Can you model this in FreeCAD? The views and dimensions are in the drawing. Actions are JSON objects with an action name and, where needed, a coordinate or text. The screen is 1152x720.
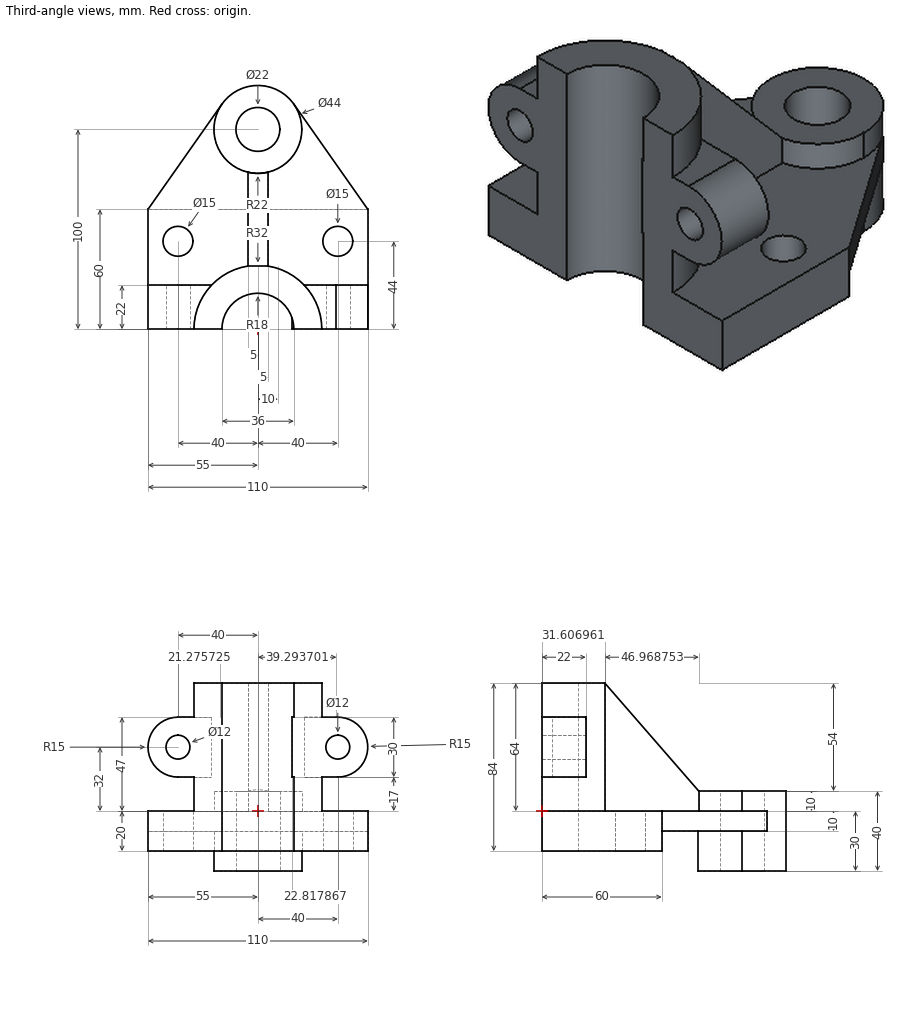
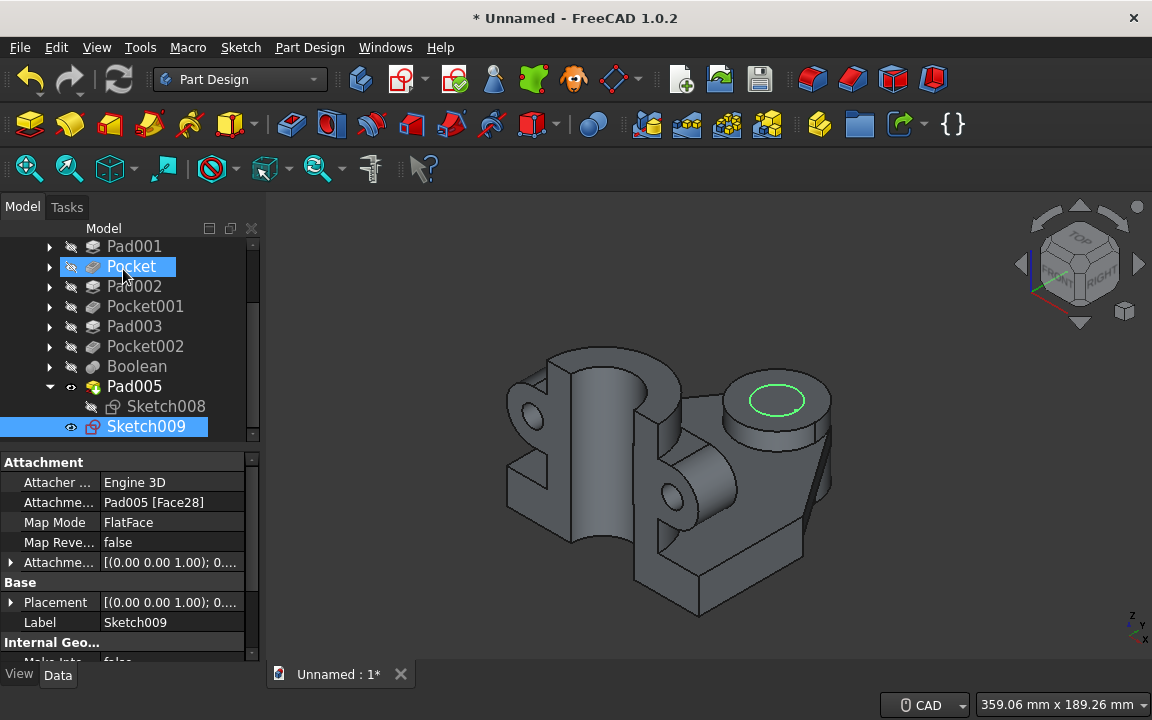
{"action": "left_click", "coordinate": [292, 124]}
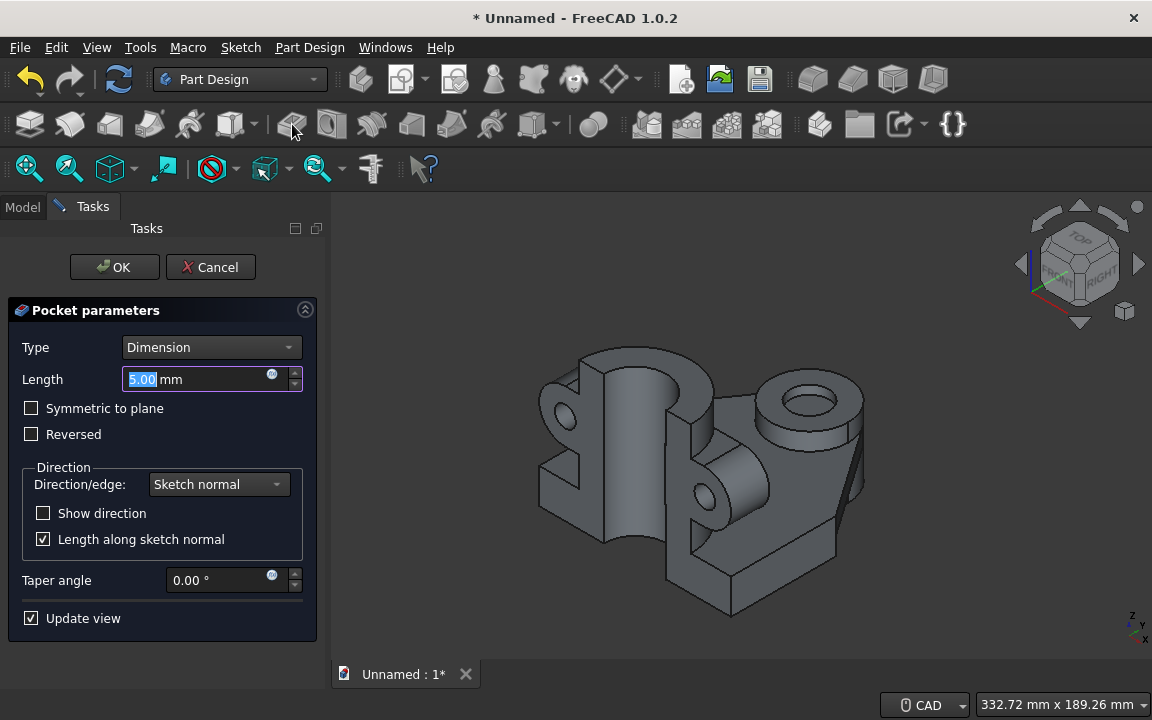
{"action": "type", "text": "40"}
{"action": "key", "text": "Tab"}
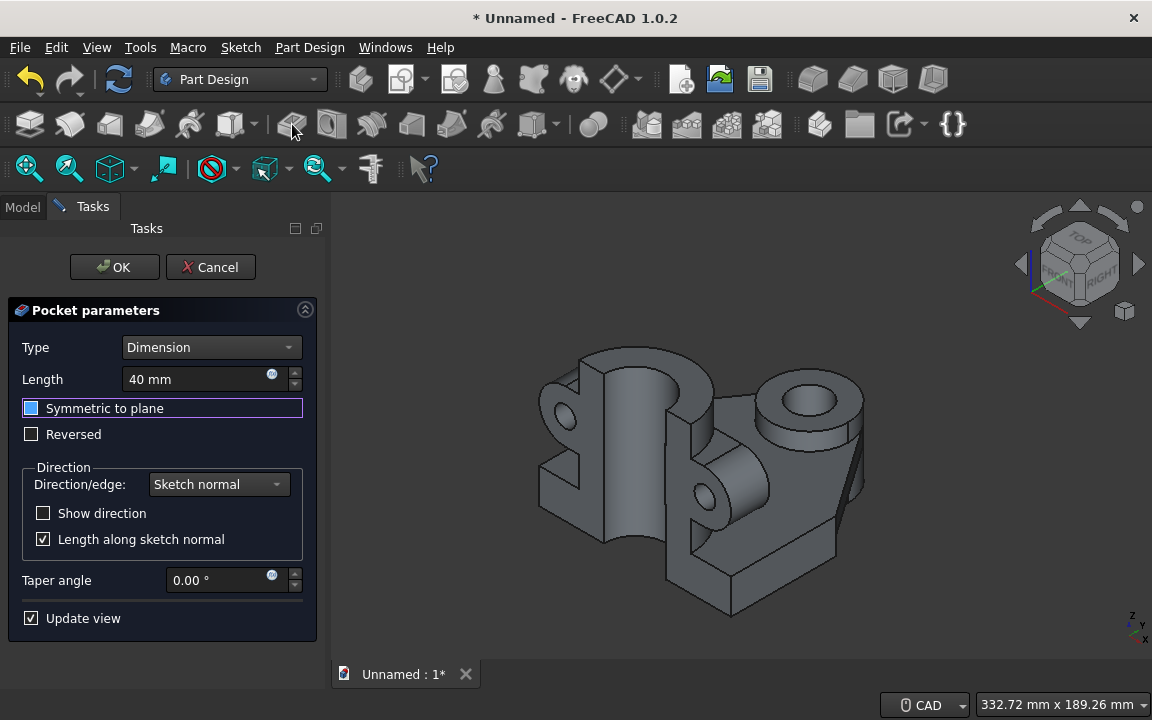
{"action": "left_click", "coordinate": [115, 267]}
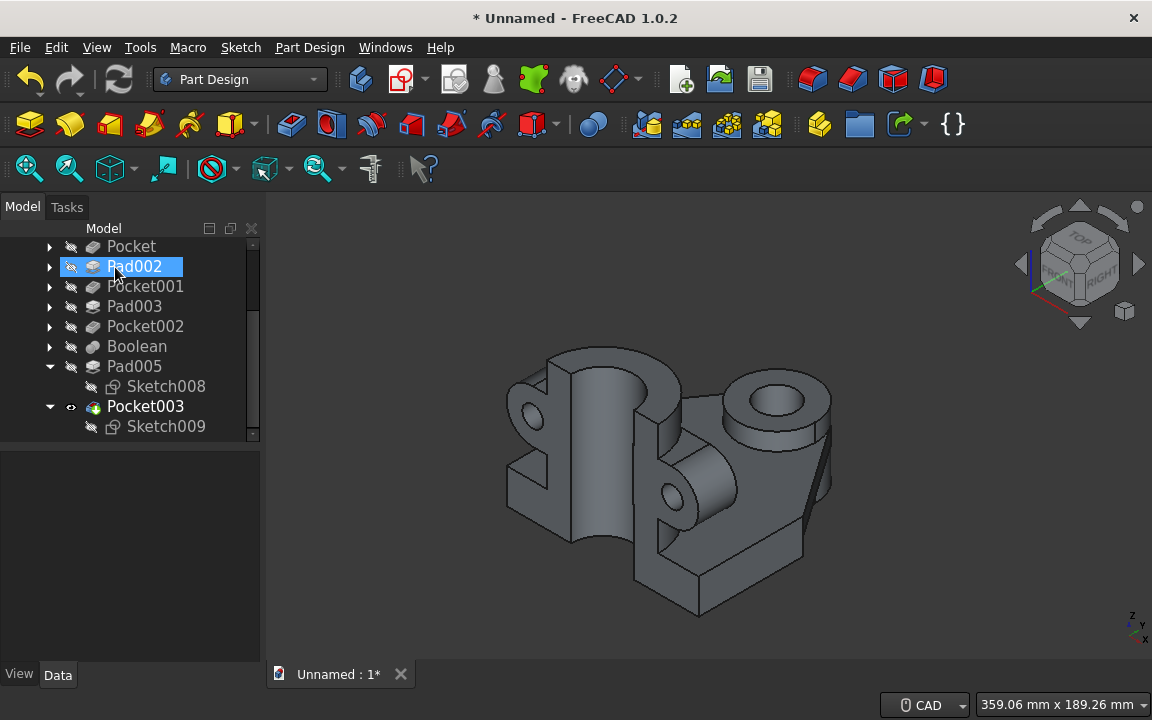
{"action": "left_click", "coordinate": [756, 495]}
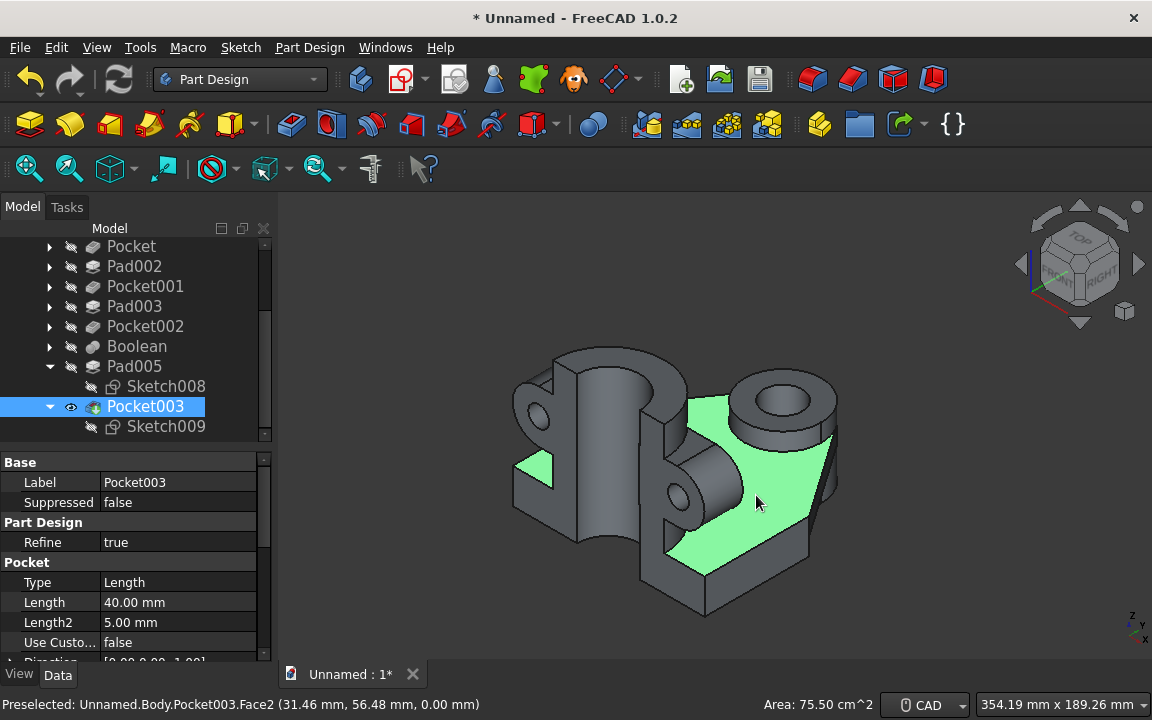
{"action": "left_click", "coordinate": [402, 80]}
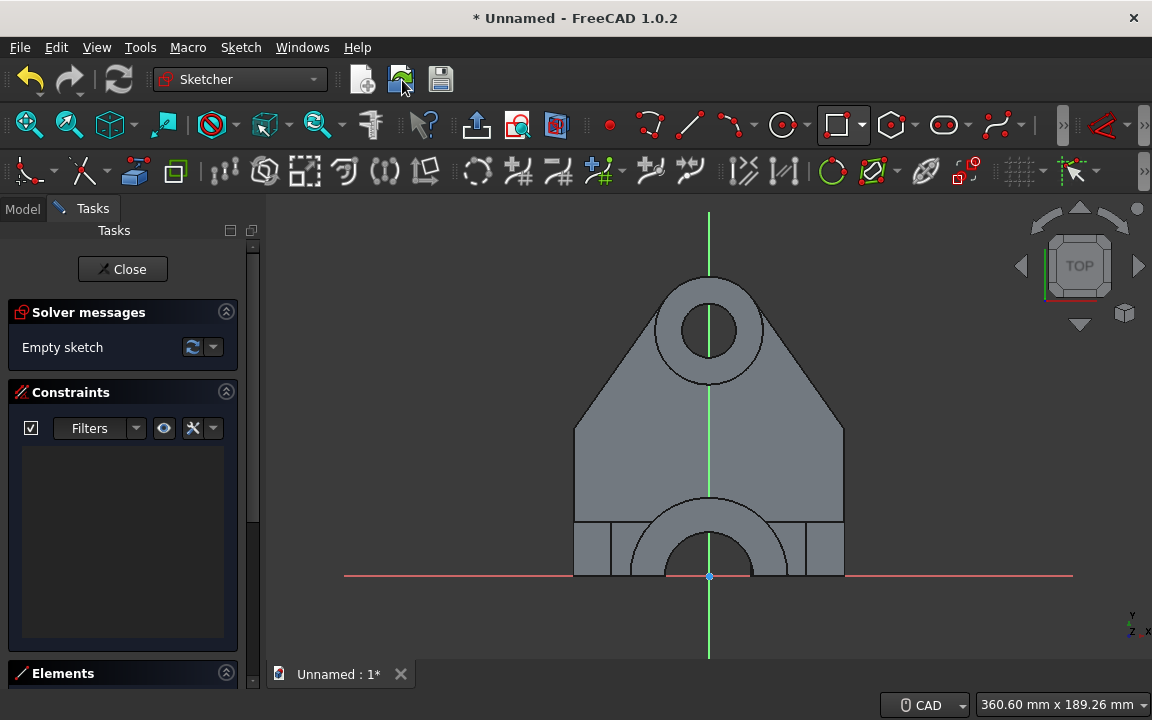
{"action": "scroll", "coordinate": [848, 588], "scroll_direction": "up", "scroll_amount": 2}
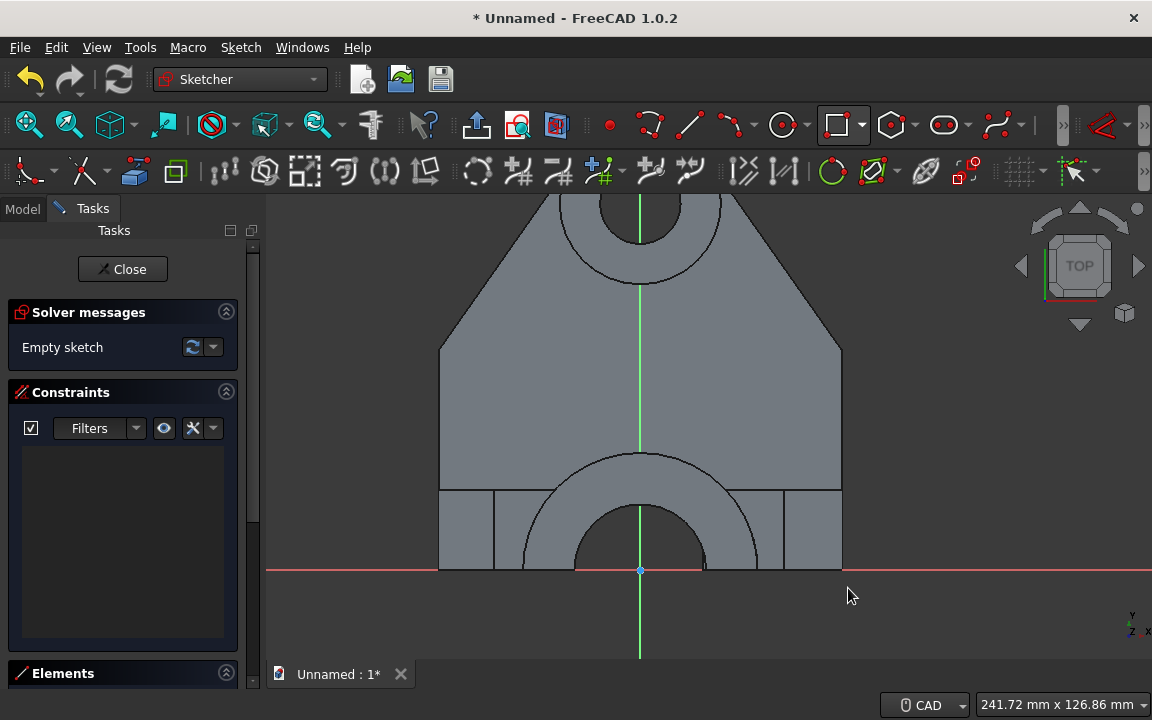
{"action": "left_click", "coordinate": [690, 126]}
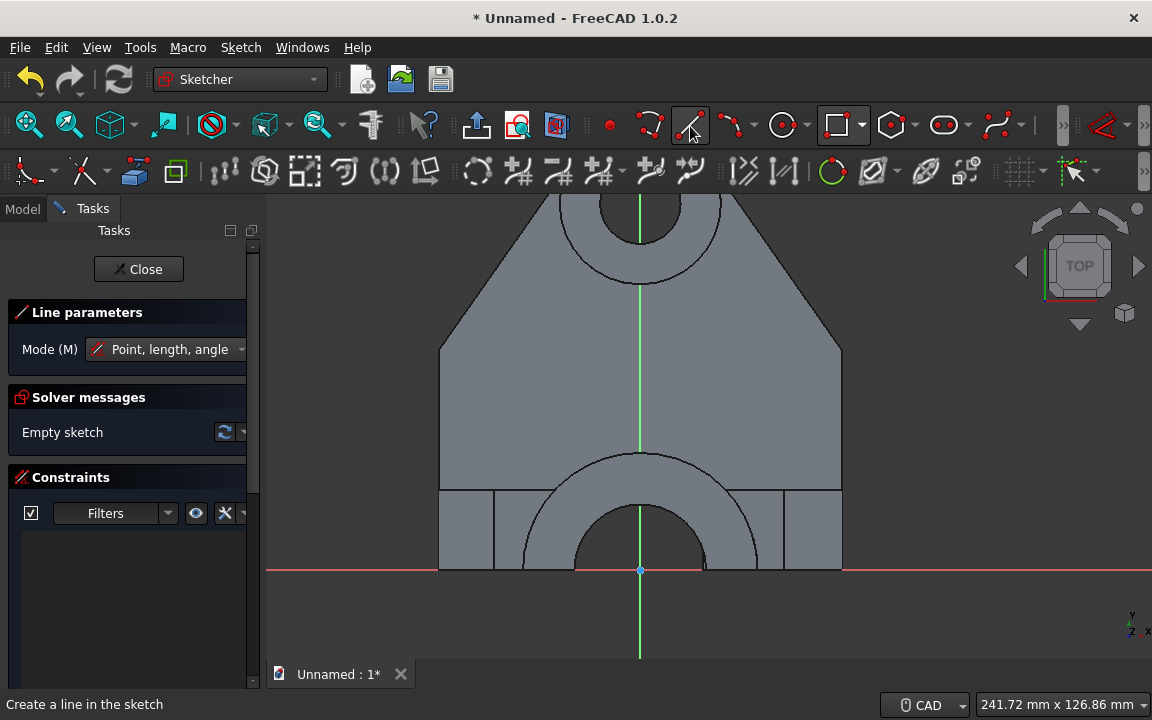
{"action": "left_click", "coordinate": [622, 282]}
{"action": "left_click", "coordinate": [622, 454]}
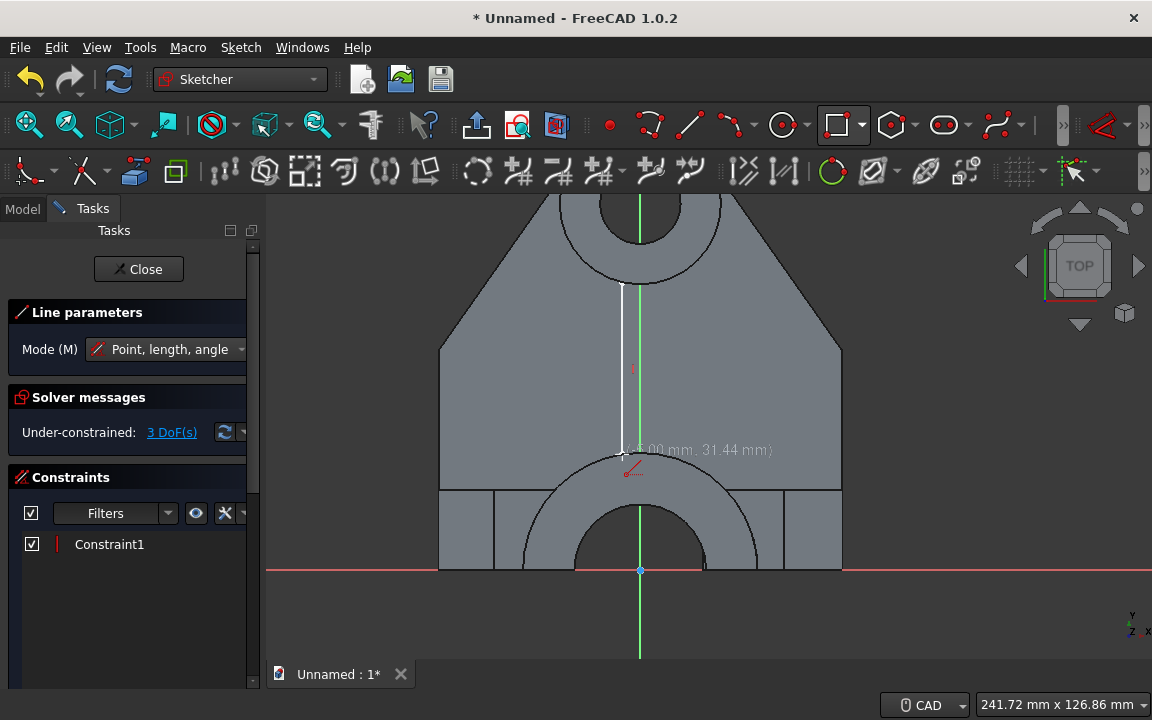
{"action": "left_click", "coordinate": [659, 454]}
{"action": "left_click", "coordinate": [659, 282]}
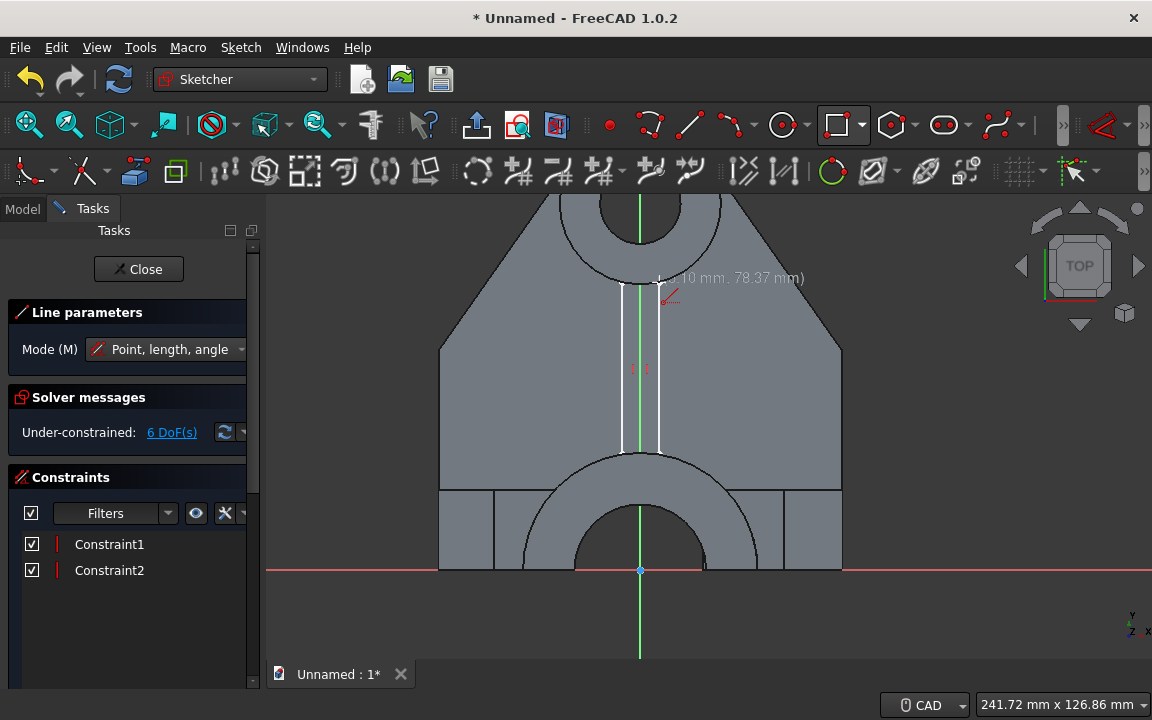
{"action": "left_click", "coordinate": [730, 126]}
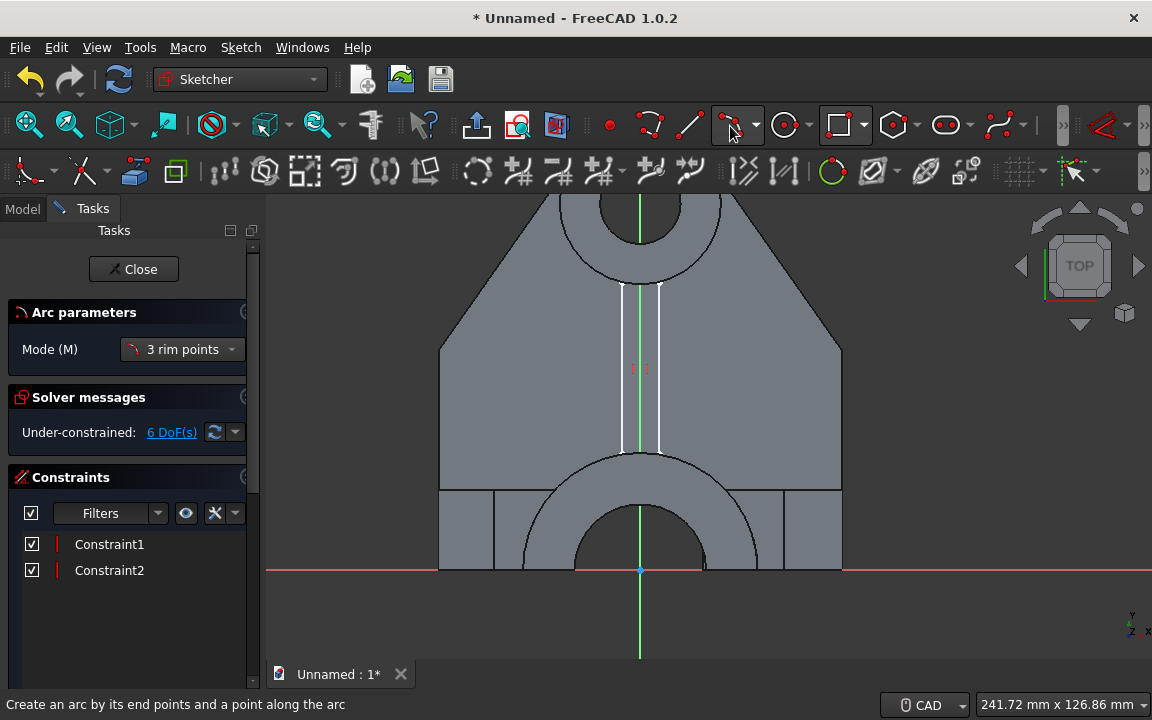
{"action": "left_click", "coordinate": [622, 455]}
{"action": "left_click", "coordinate": [659, 455]}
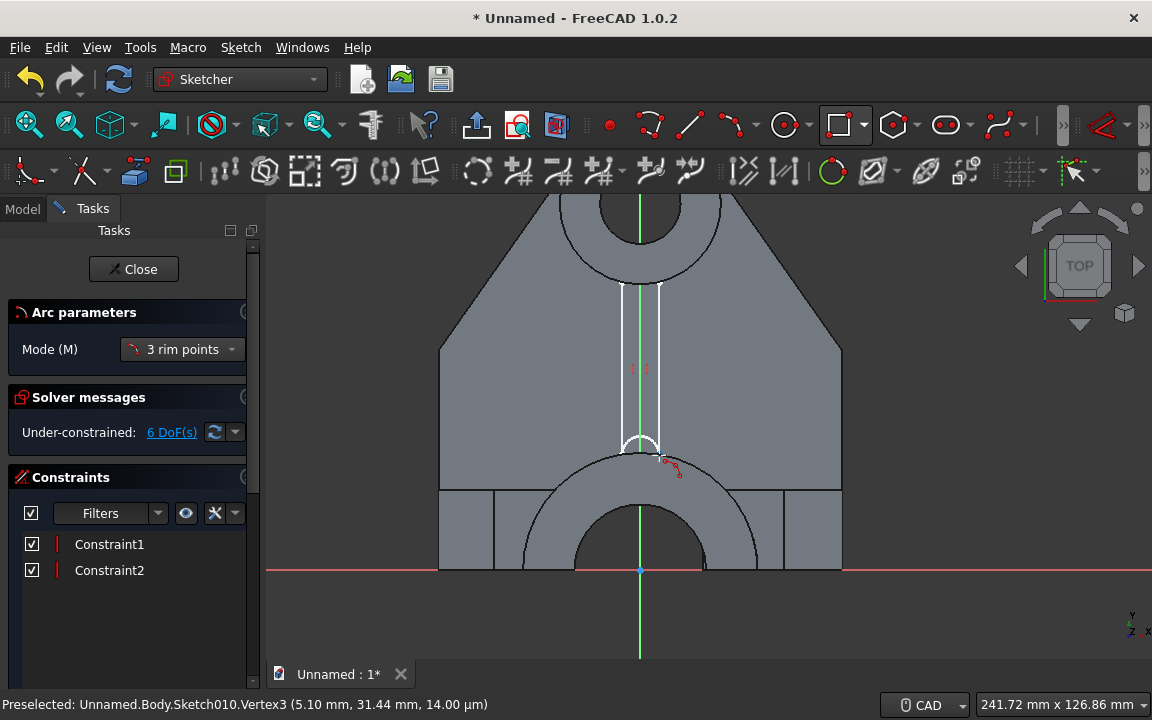
{"action": "scroll", "coordinate": [644, 453], "scroll_direction": "up", "scroll_amount": 13}